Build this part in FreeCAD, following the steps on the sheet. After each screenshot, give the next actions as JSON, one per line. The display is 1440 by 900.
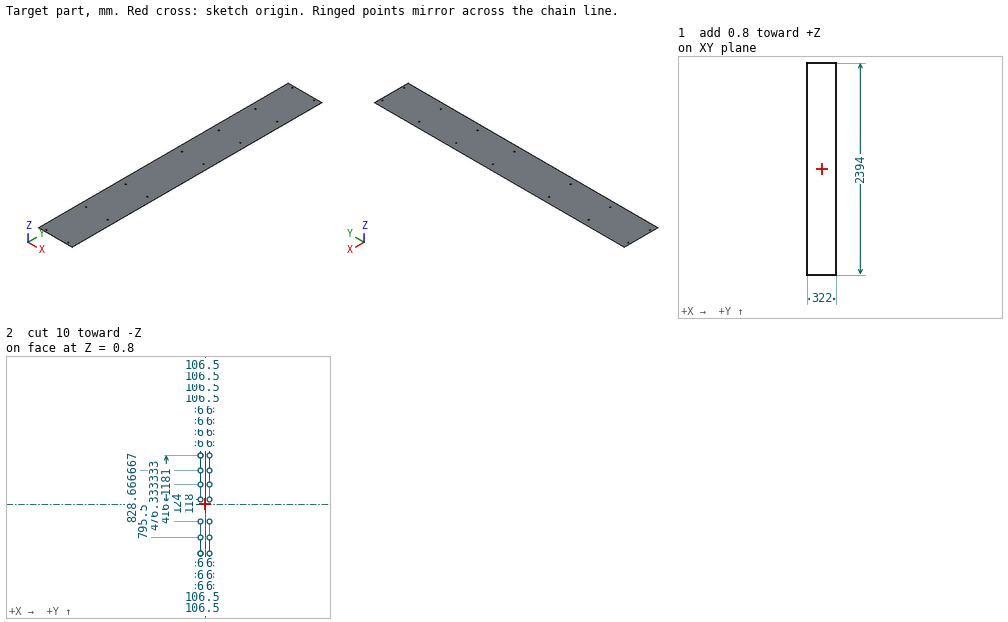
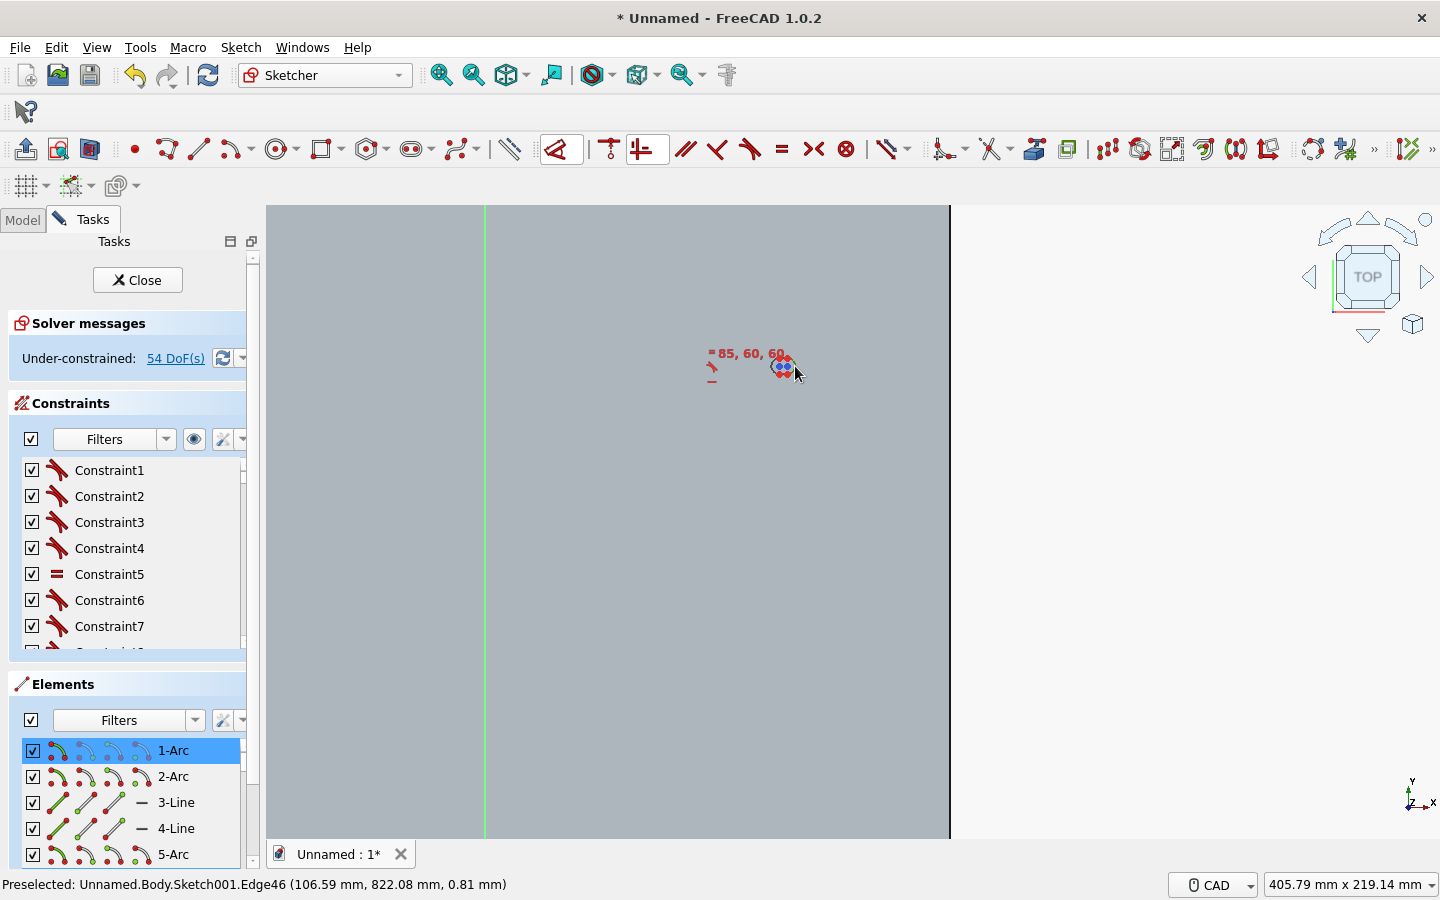
{"action": "left_click", "coordinate": [782, 150]}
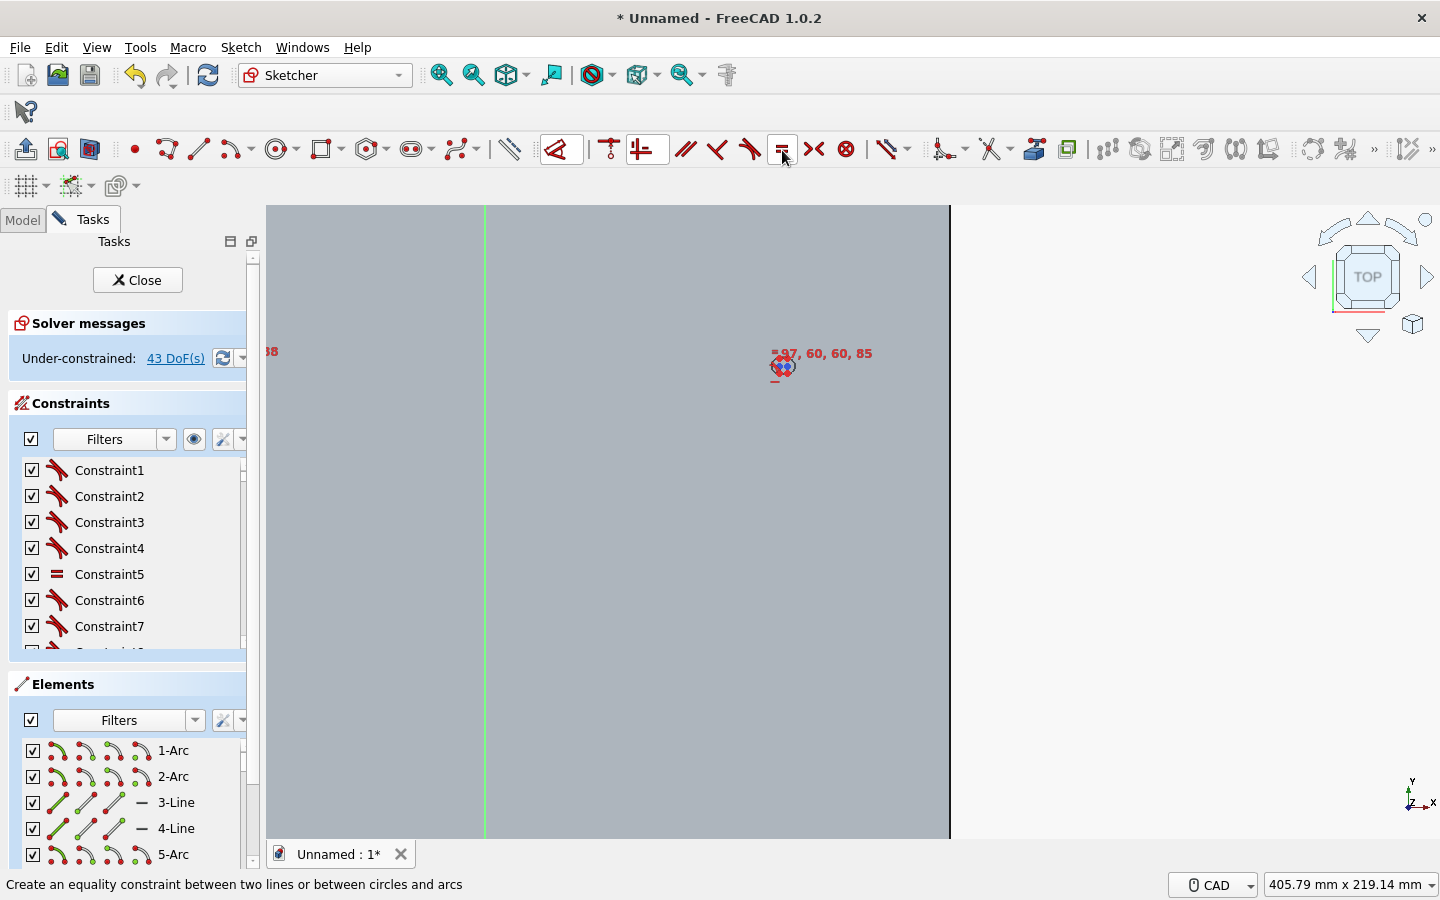
{"action": "scroll", "coordinate": [804, 378], "scroll_direction": "down", "scroll_amount": 14}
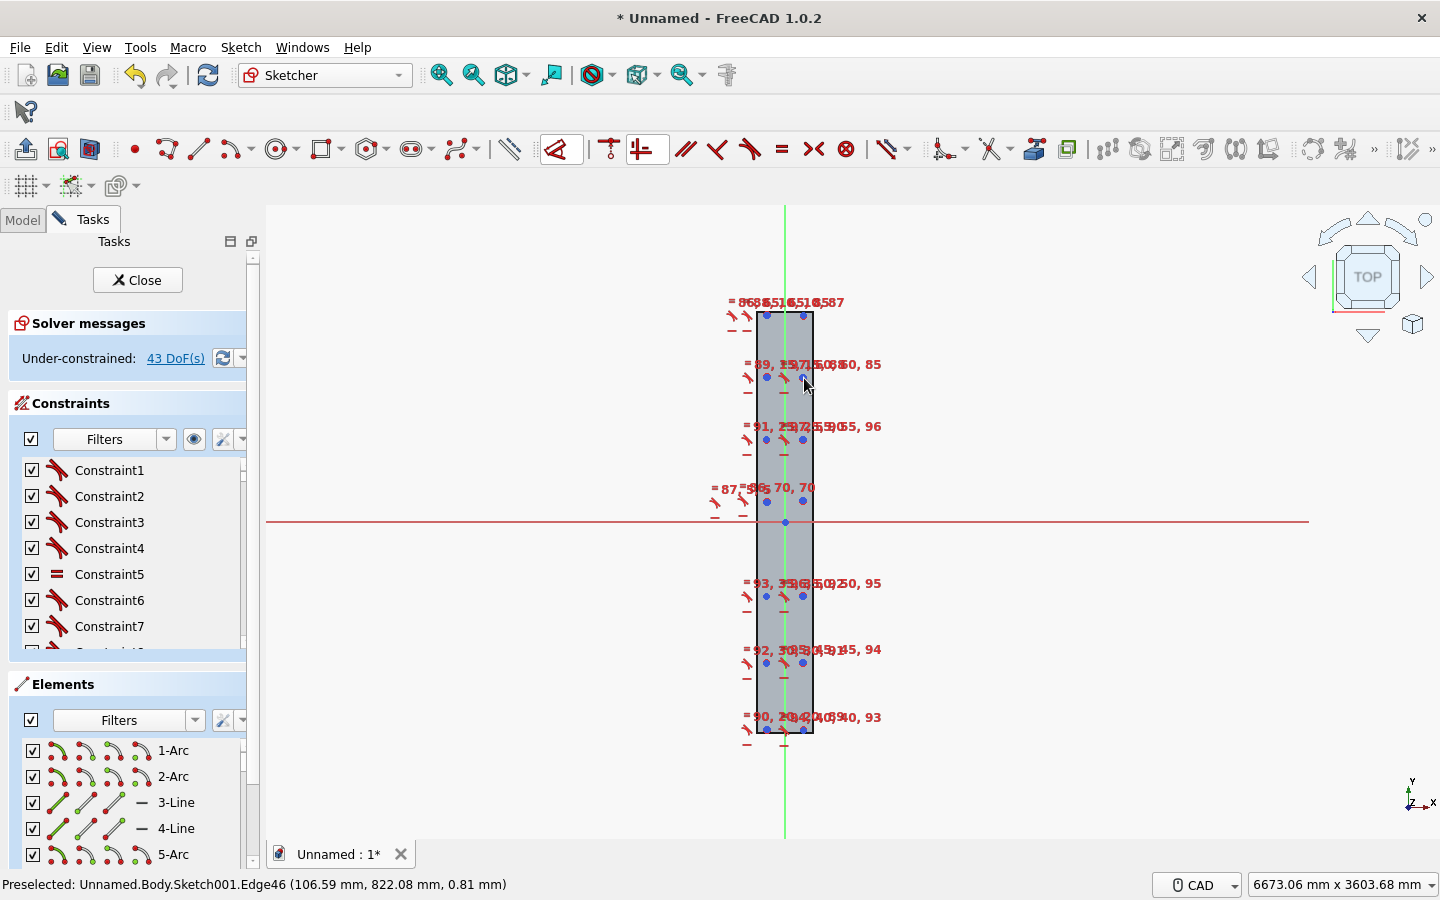
{"action": "scroll", "coordinate": [766, 315], "scroll_direction": "up", "scroll_amount": 14}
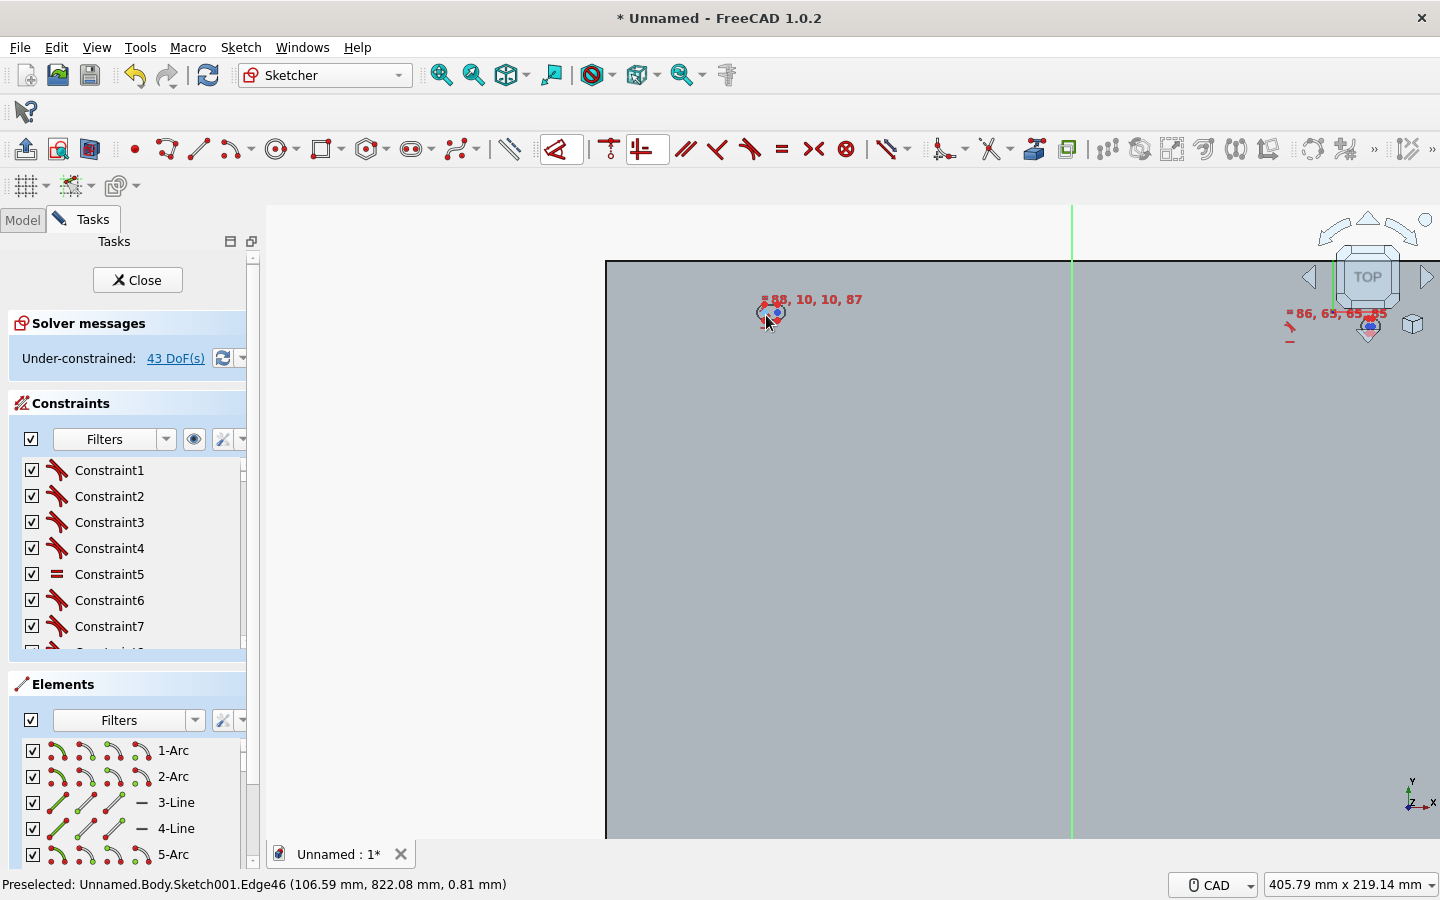
{"action": "left_click", "coordinate": [765, 312]}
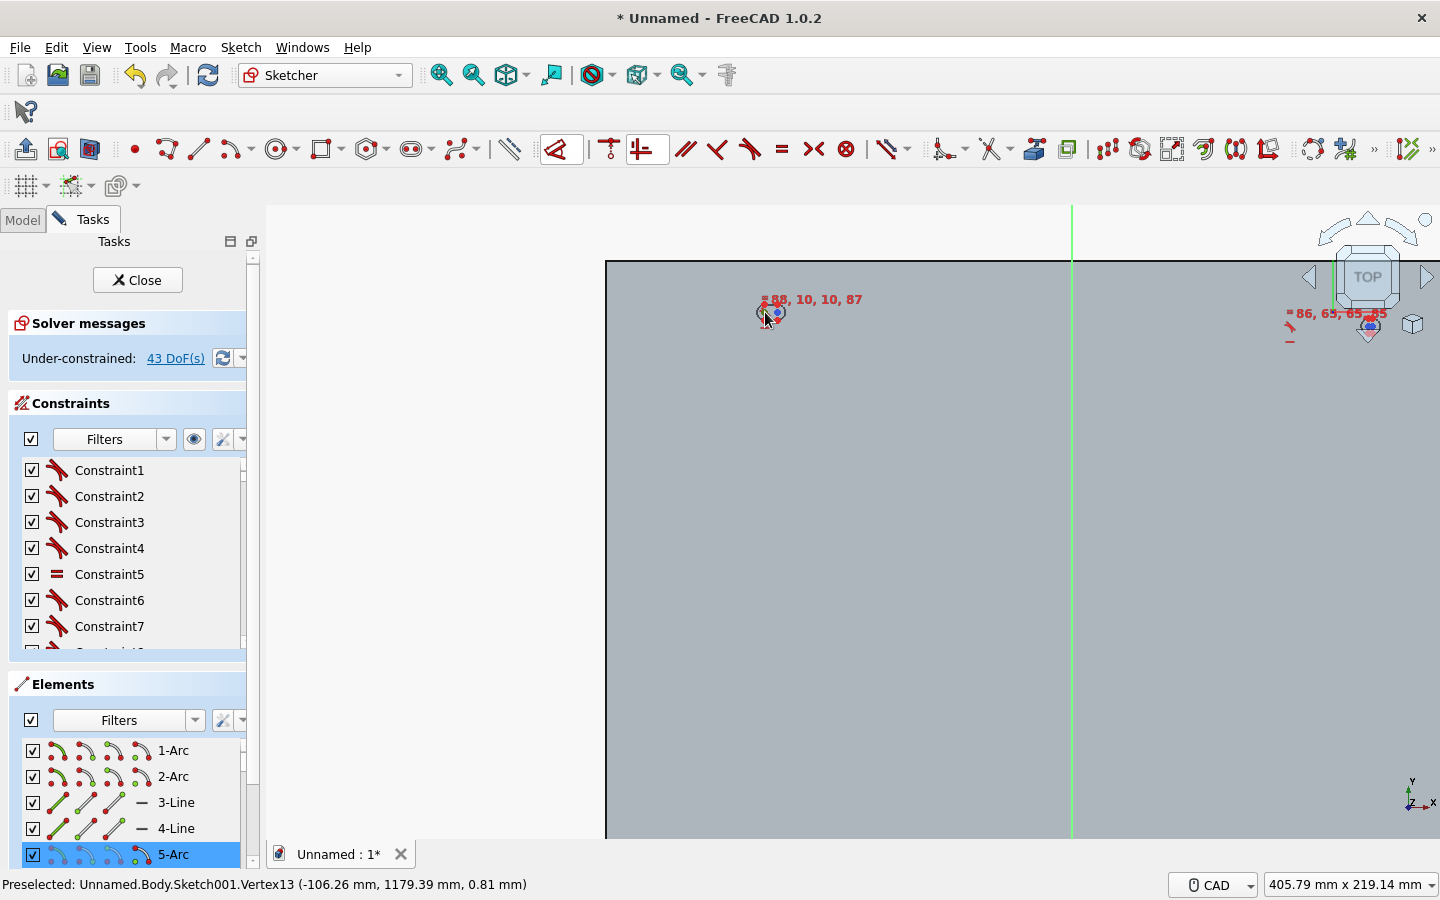
{"action": "scroll", "coordinate": [766, 315], "scroll_direction": "down", "scroll_amount": 14}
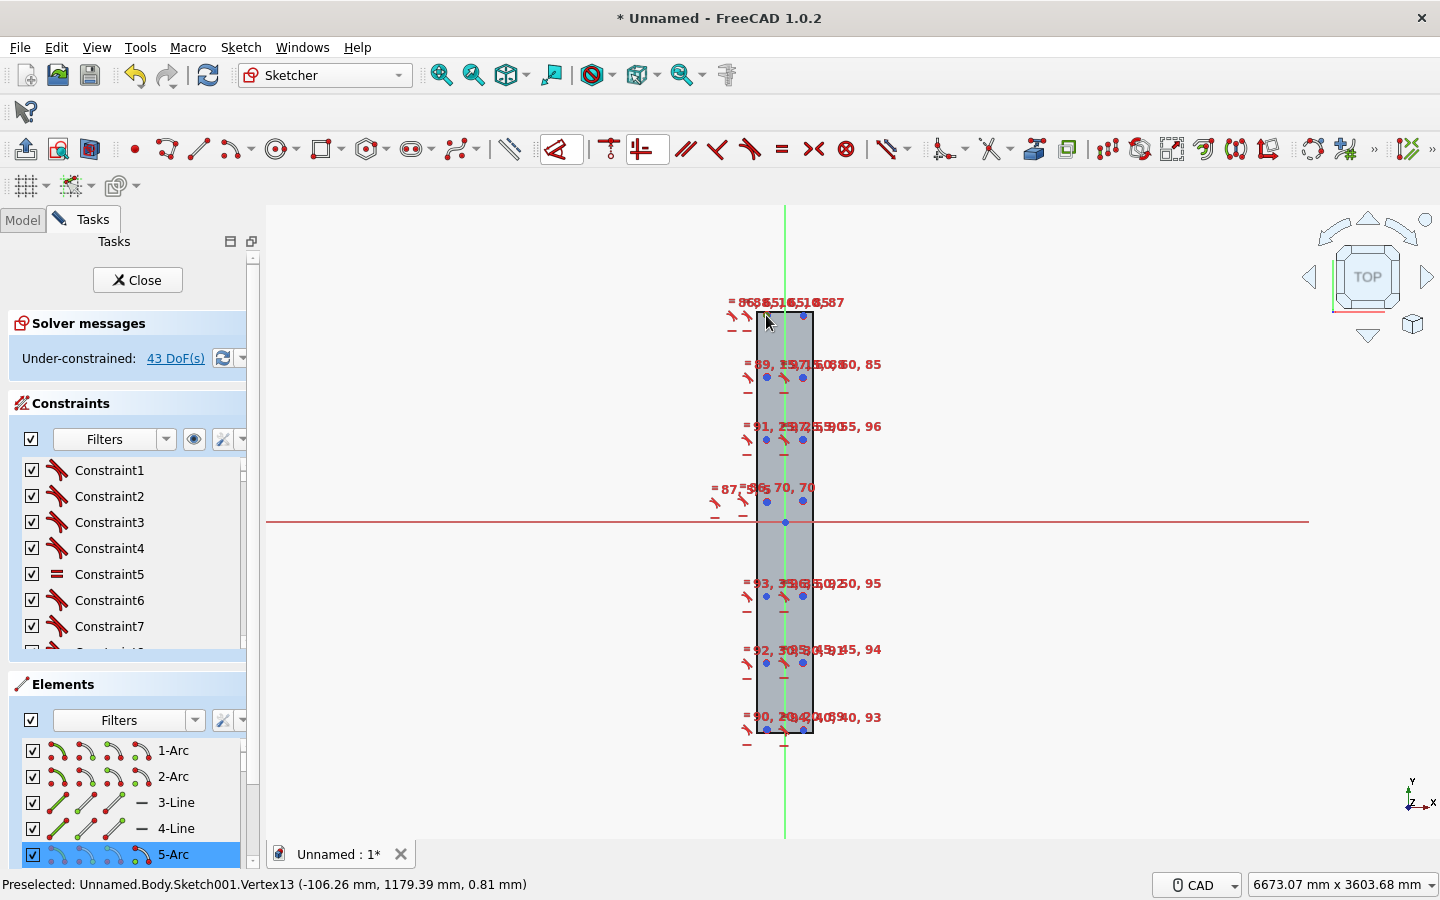
{"action": "scroll", "coordinate": [766, 730], "scroll_direction": "up", "scroll_amount": 14}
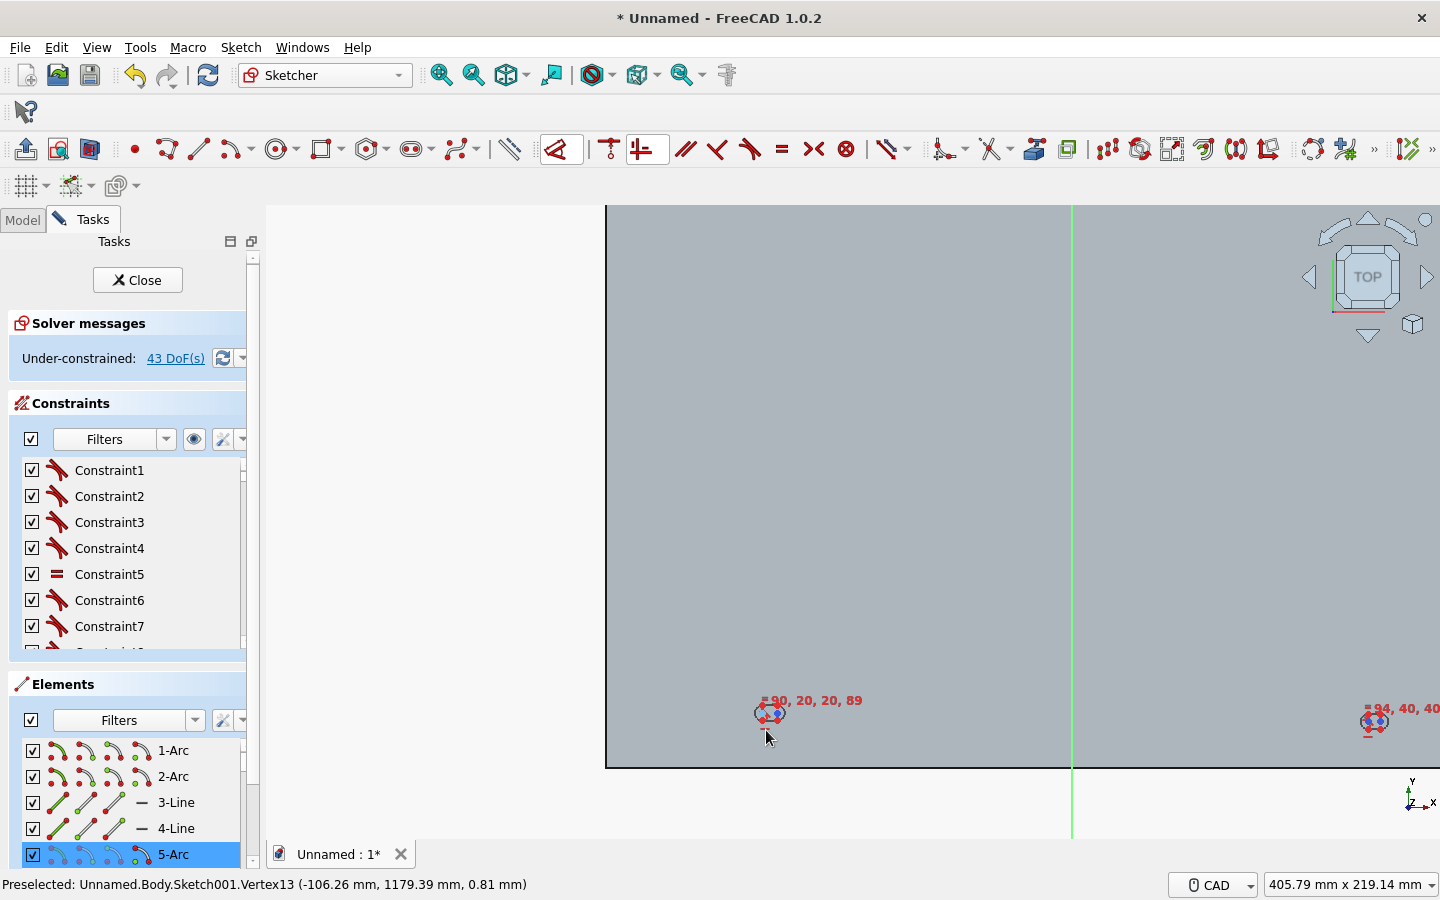
{"action": "left_click", "coordinate": [763, 713]}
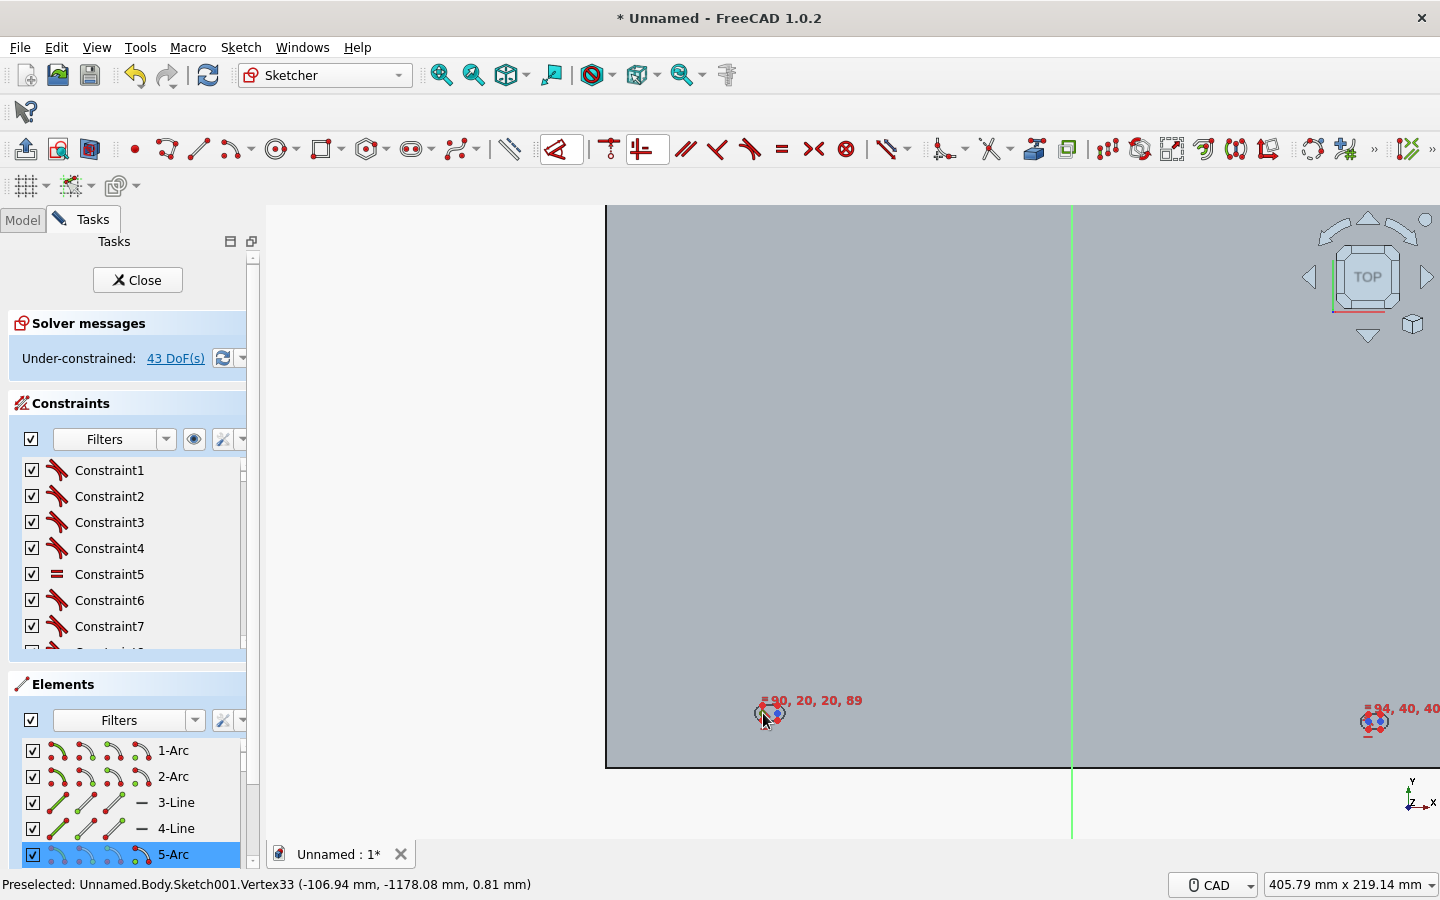
{"action": "scroll", "coordinate": [766, 730], "scroll_direction": "down", "scroll_amount": 14}